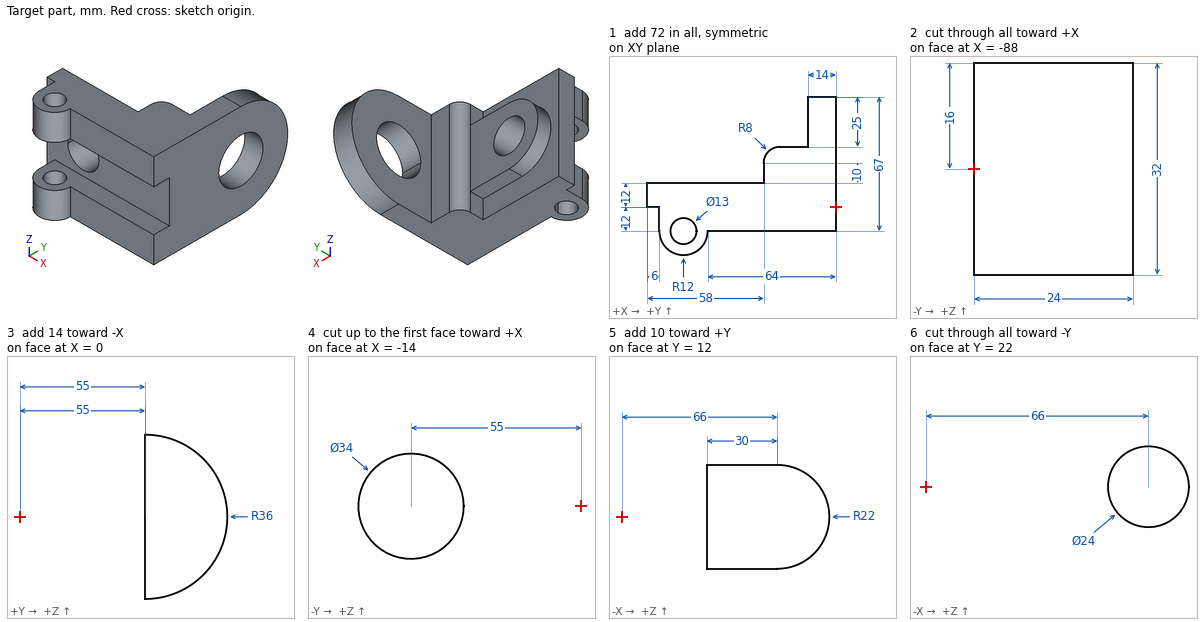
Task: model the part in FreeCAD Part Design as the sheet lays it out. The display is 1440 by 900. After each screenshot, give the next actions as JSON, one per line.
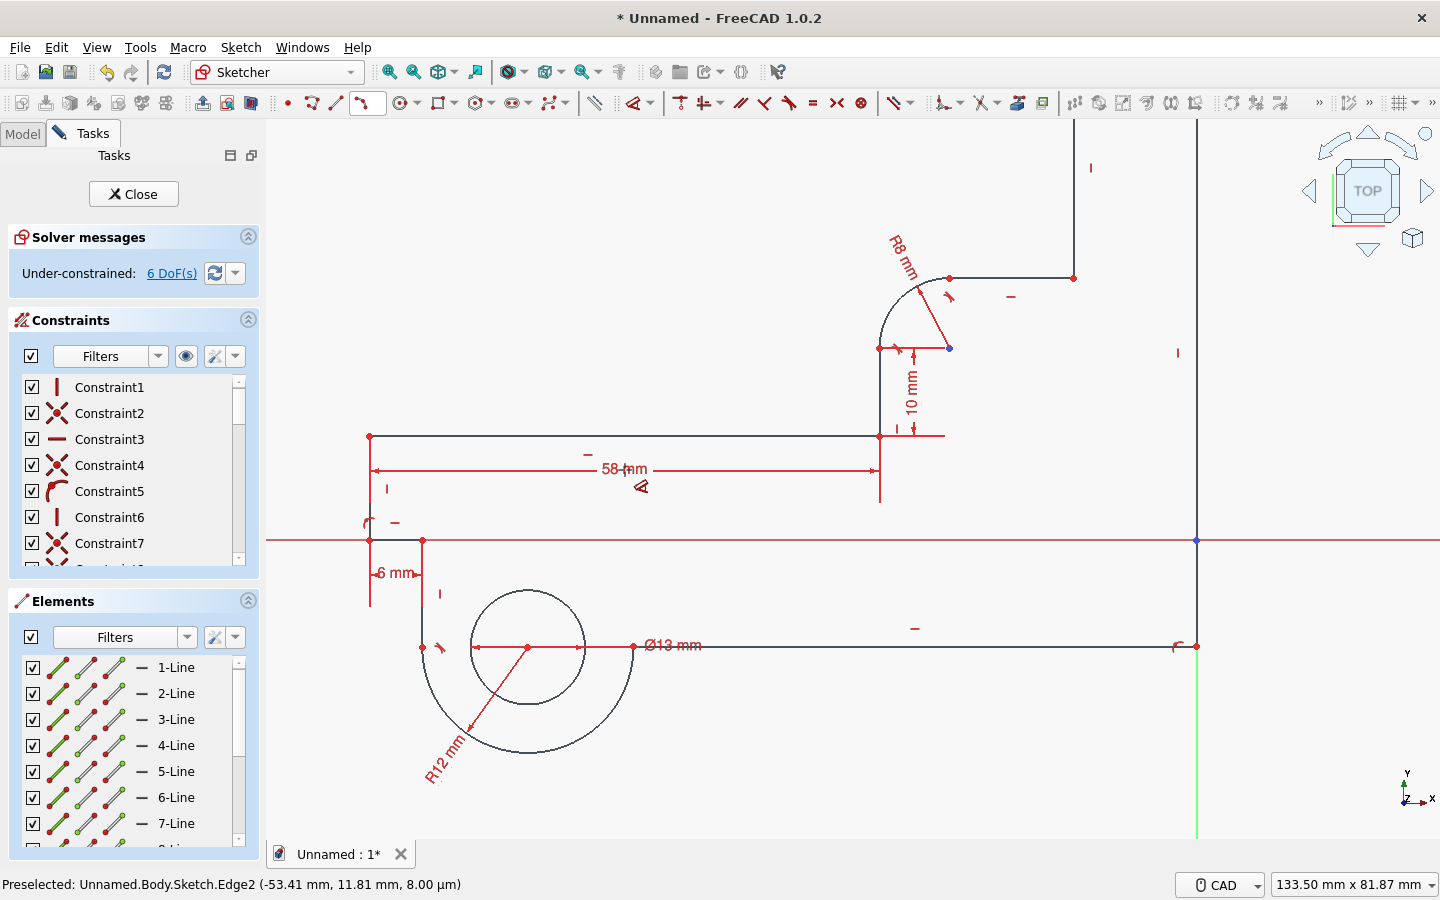
{"action": "left_click", "coordinate": [370, 468]}
{"action": "left_click", "coordinate": [336, 488]}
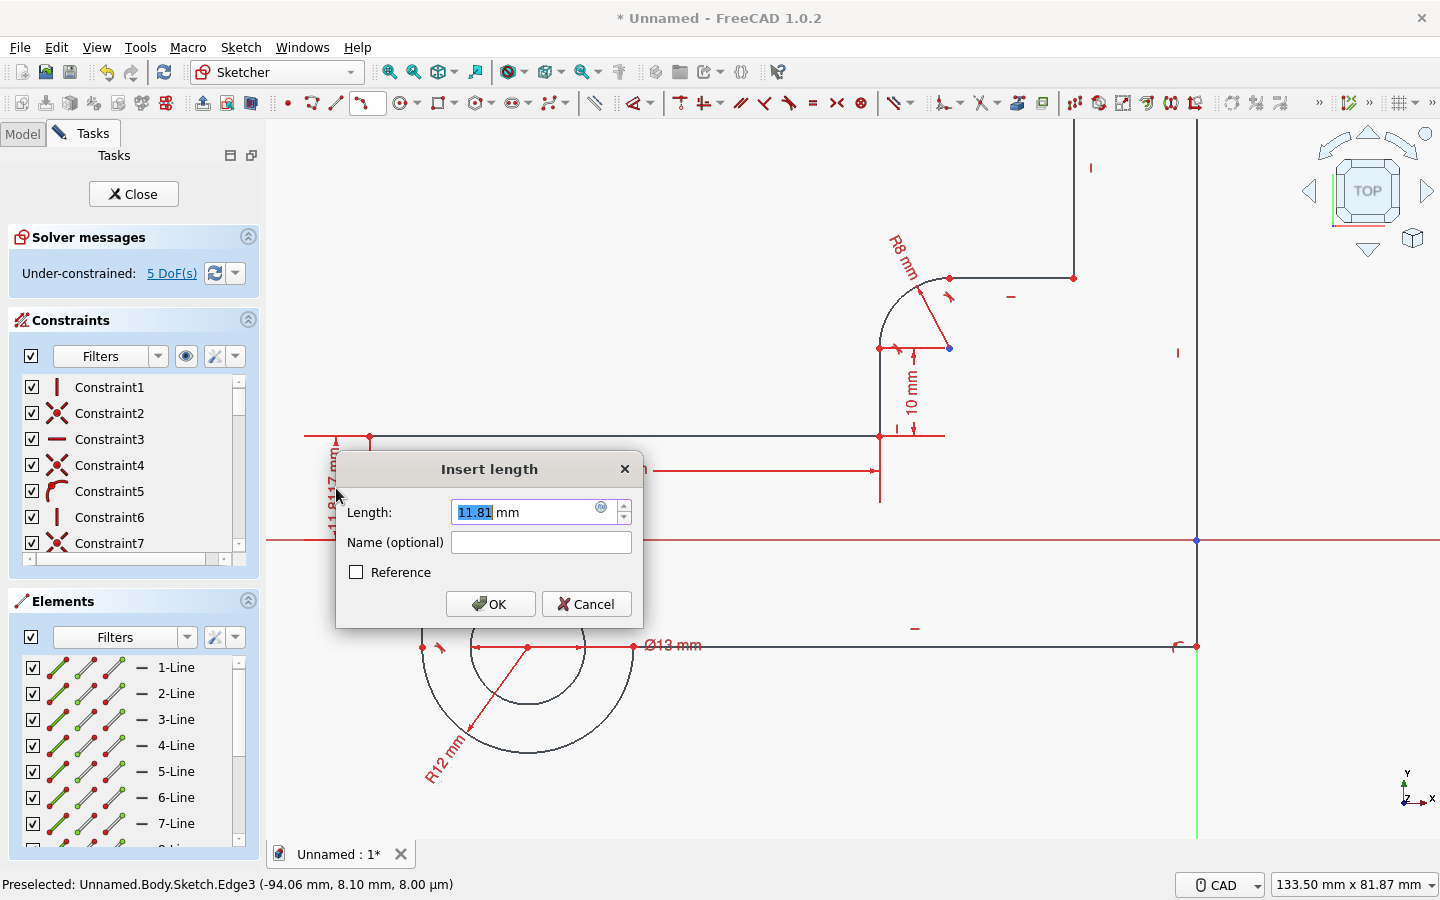
{"action": "type", "text": "12"}
{"action": "key", "text": "Return"}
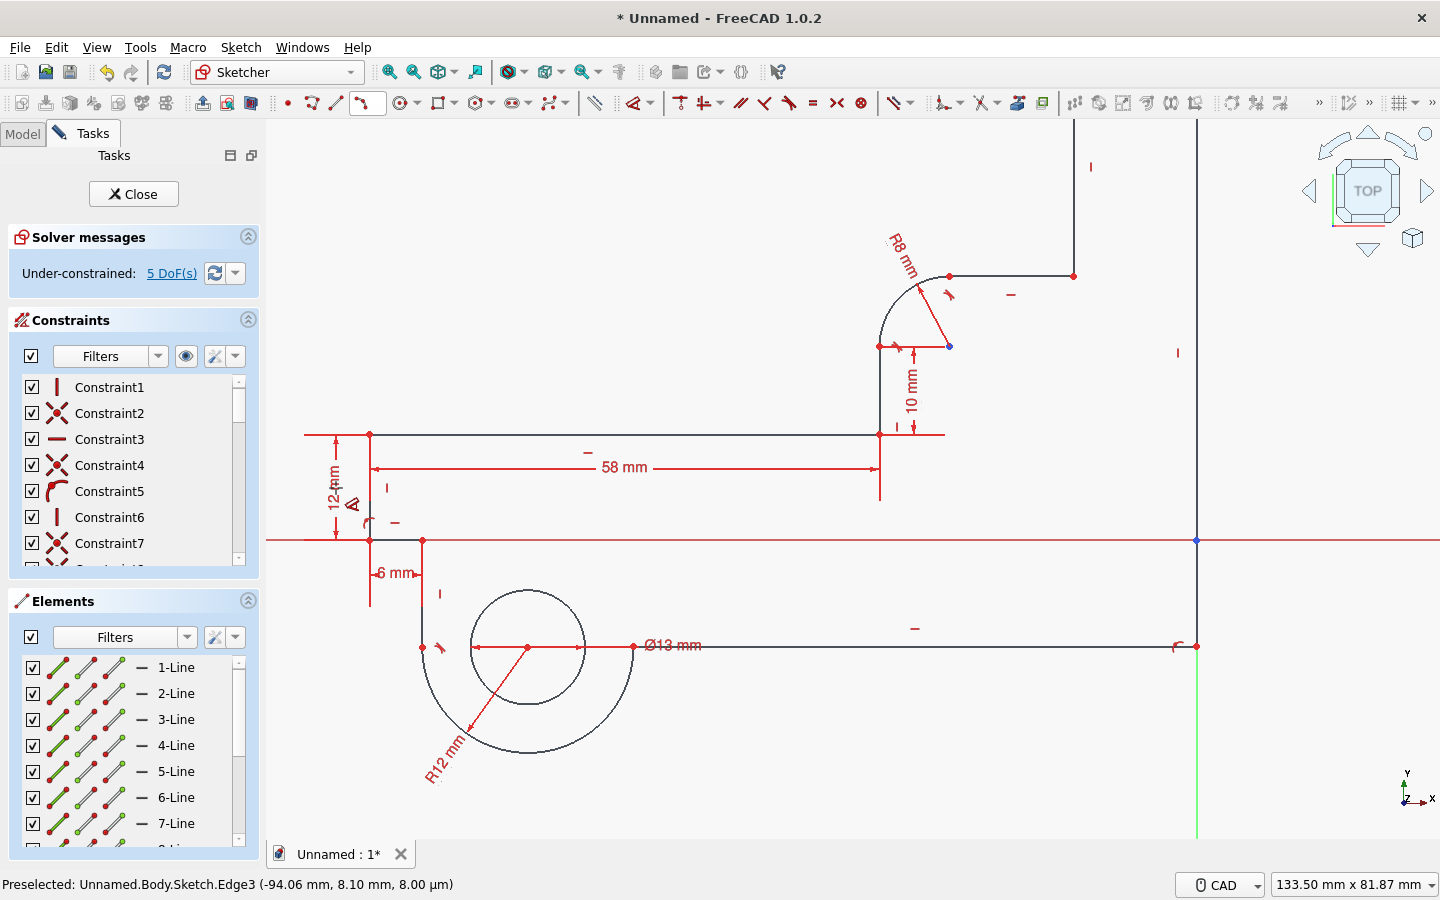
{"action": "left_click", "coordinate": [422, 572]}
{"action": "left_click", "coordinate": [388, 618]}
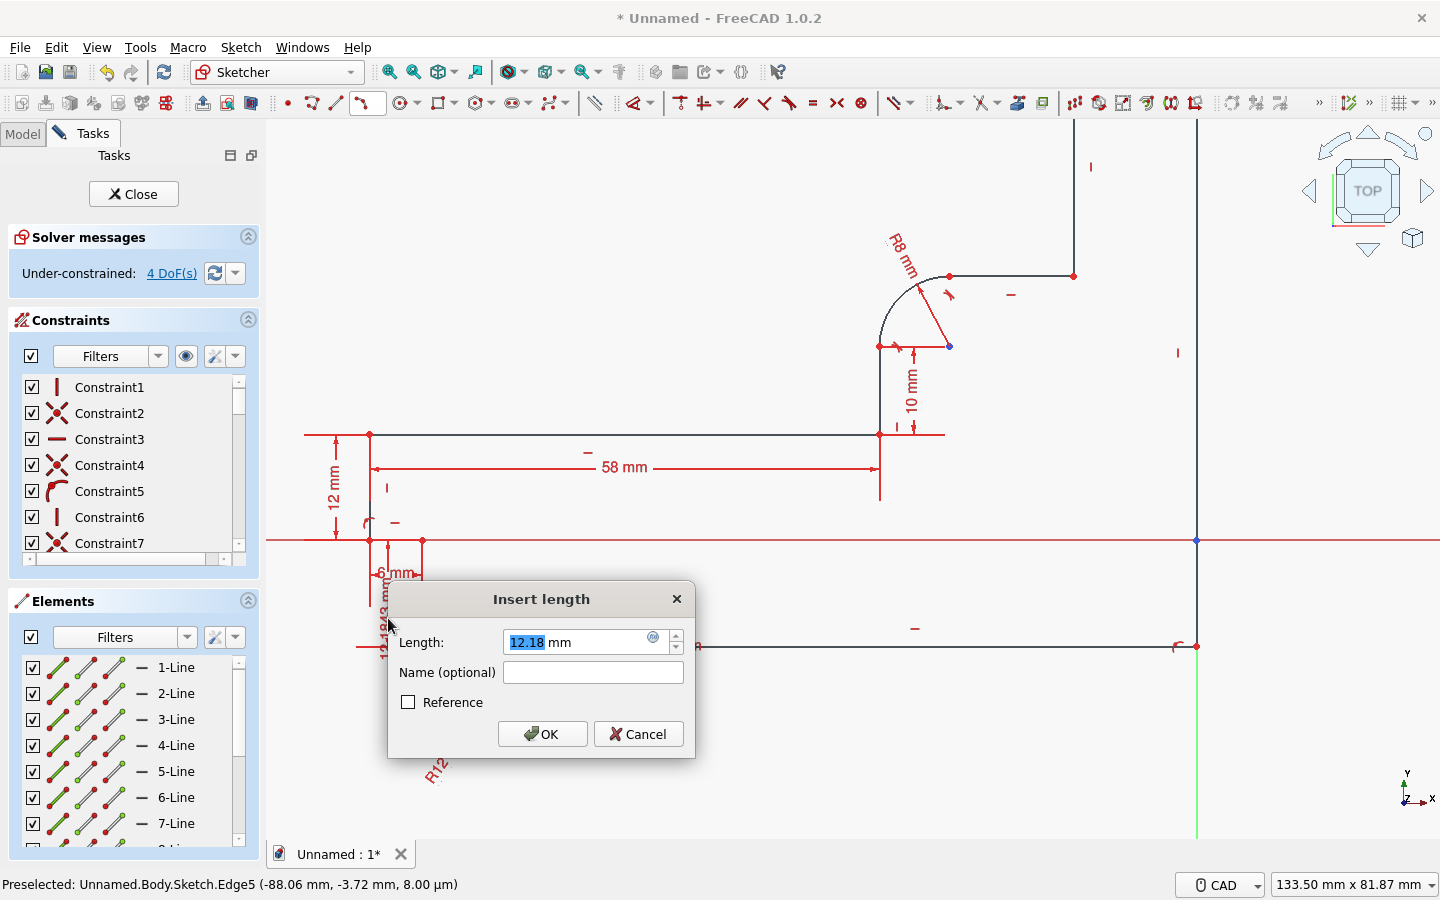
{"action": "type", "text": "12"}
{"action": "key", "text": "Return"}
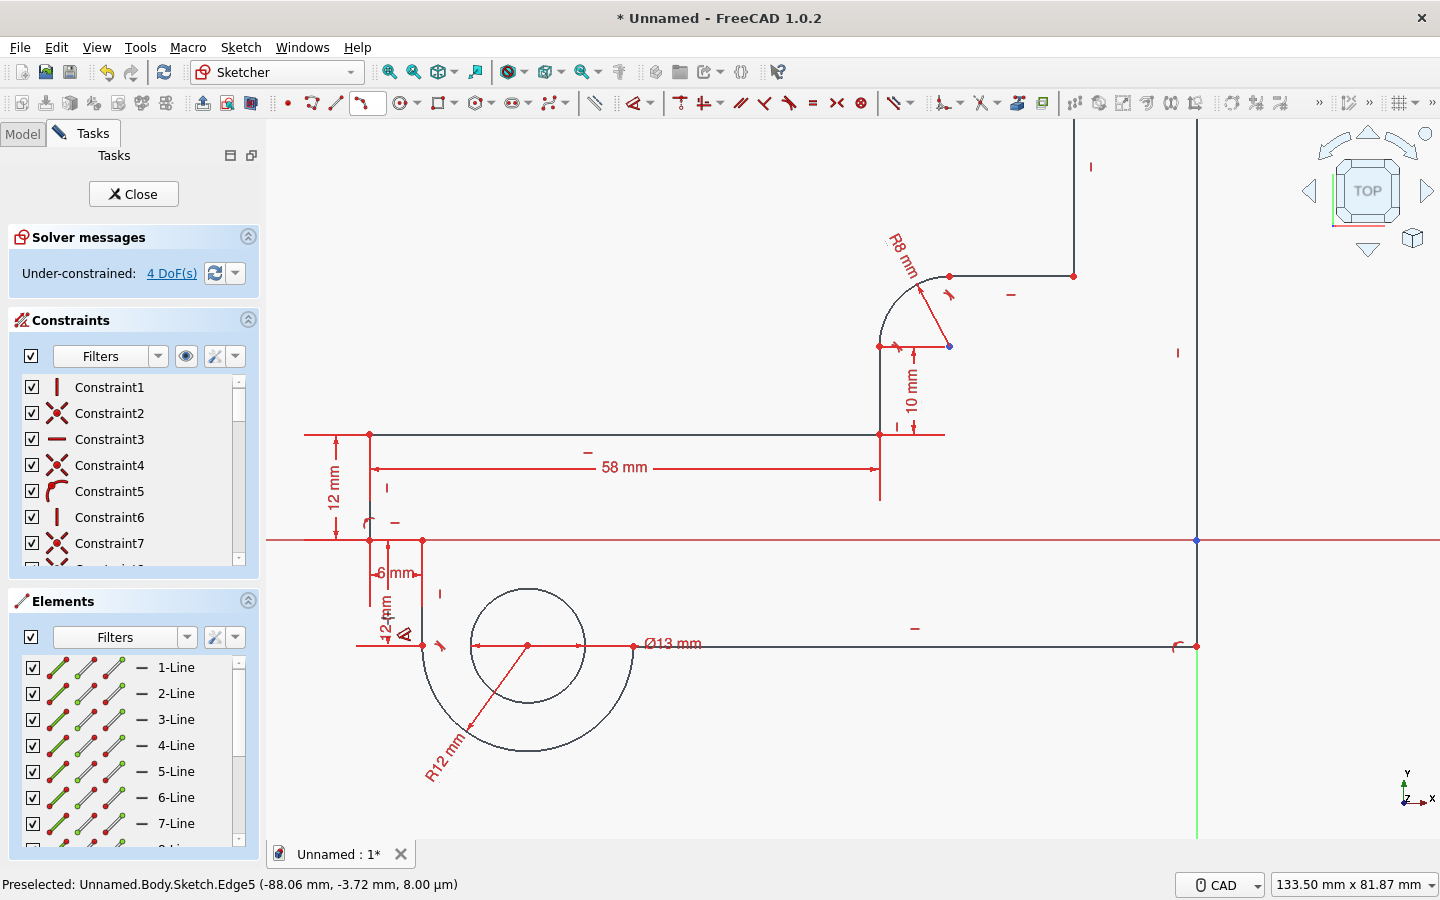
{"action": "left_click", "coordinate": [802, 647]}
{"action": "left_click", "coordinate": [915, 681]}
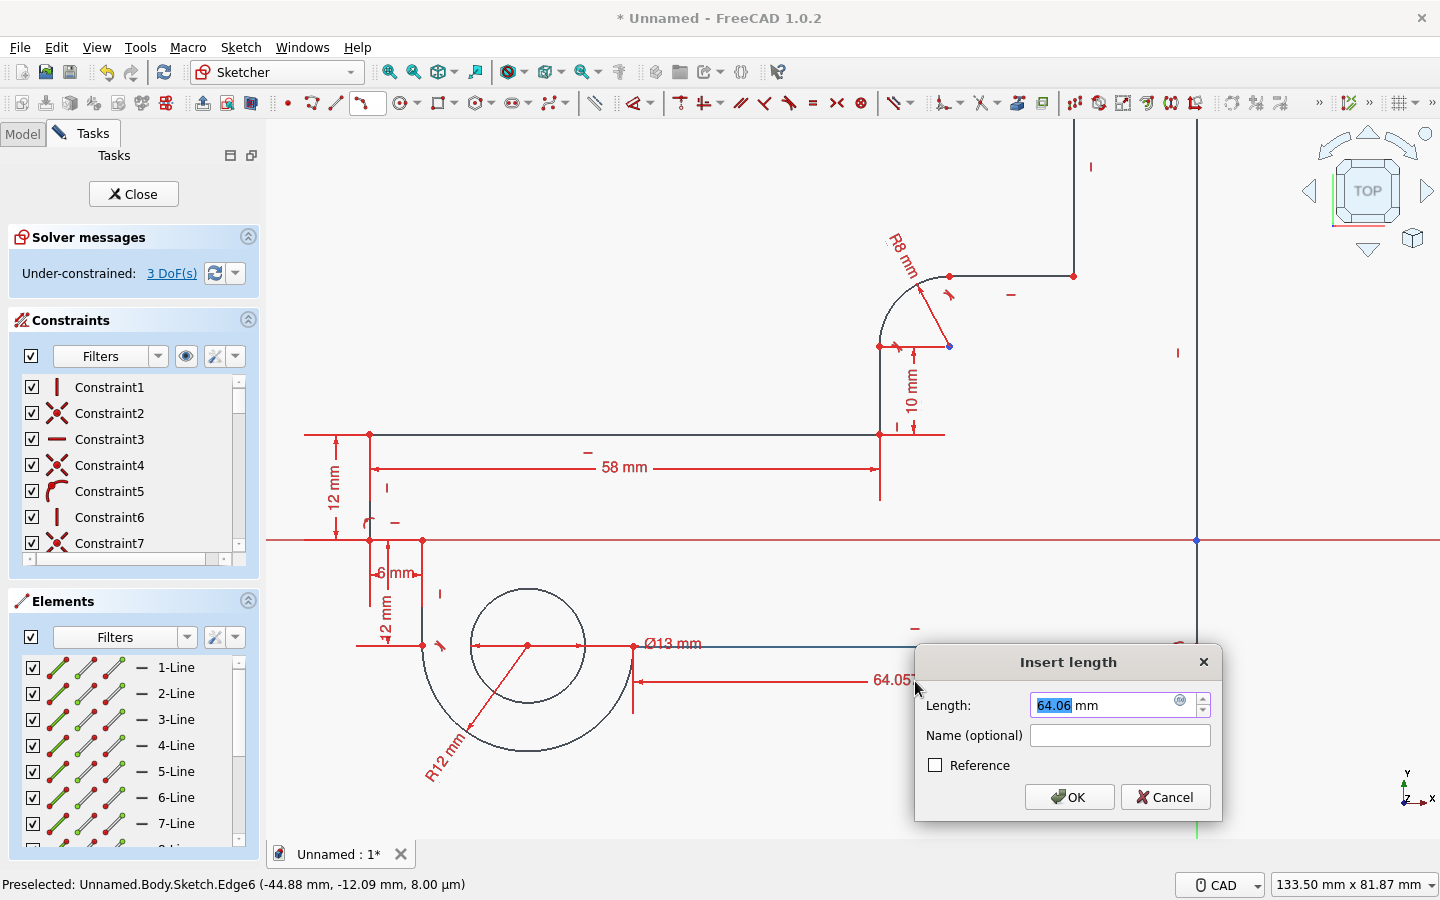
{"action": "type", "text": "64"}
{"action": "key", "text": "Return"}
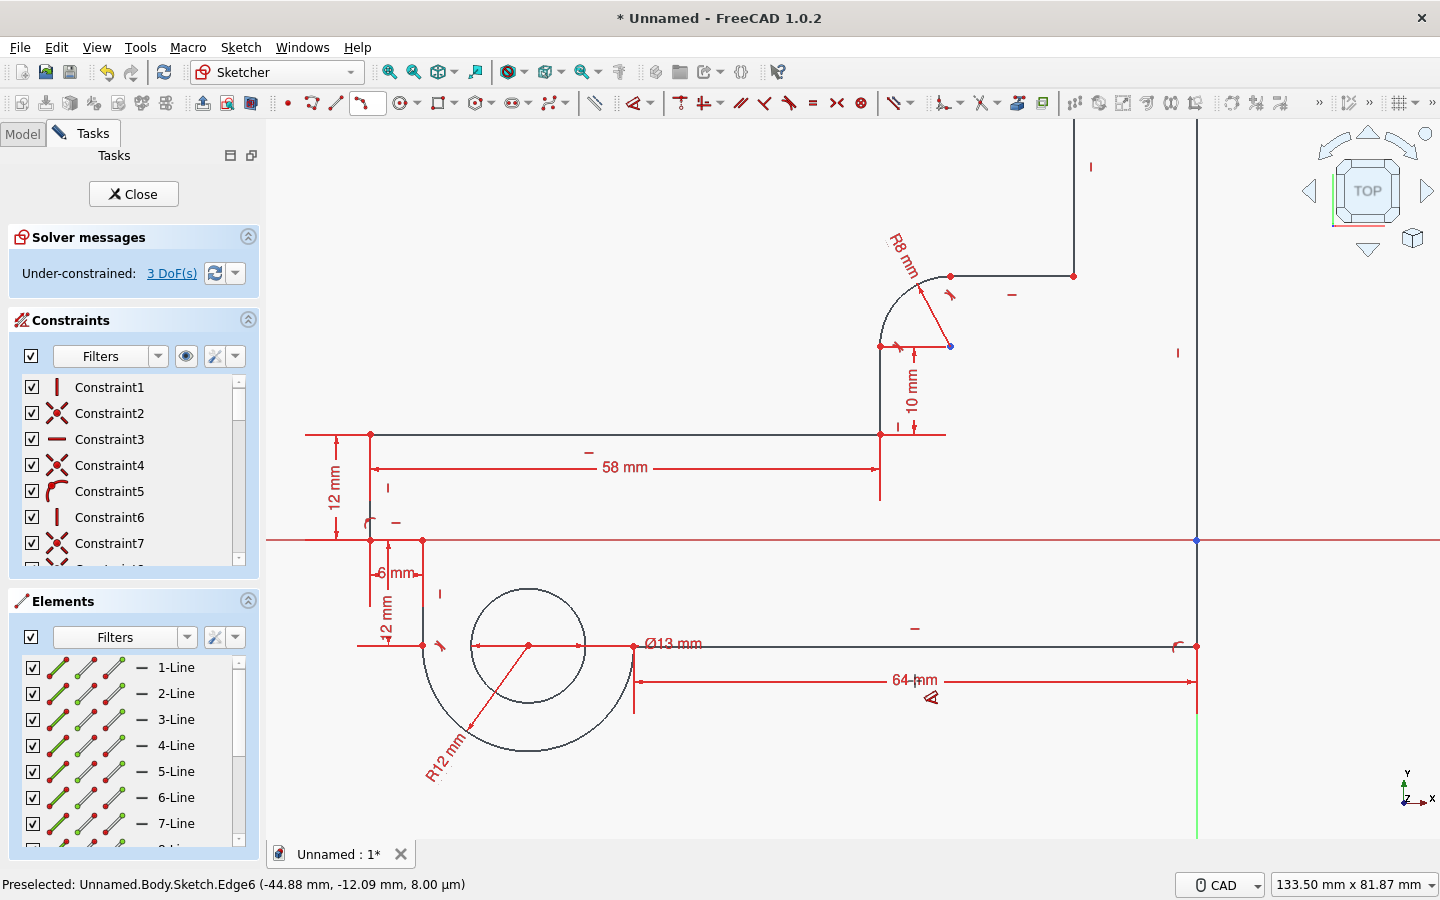
{"action": "left_click", "coordinate": [1197, 470]}
{"action": "left_click", "coordinate": [1231, 397]}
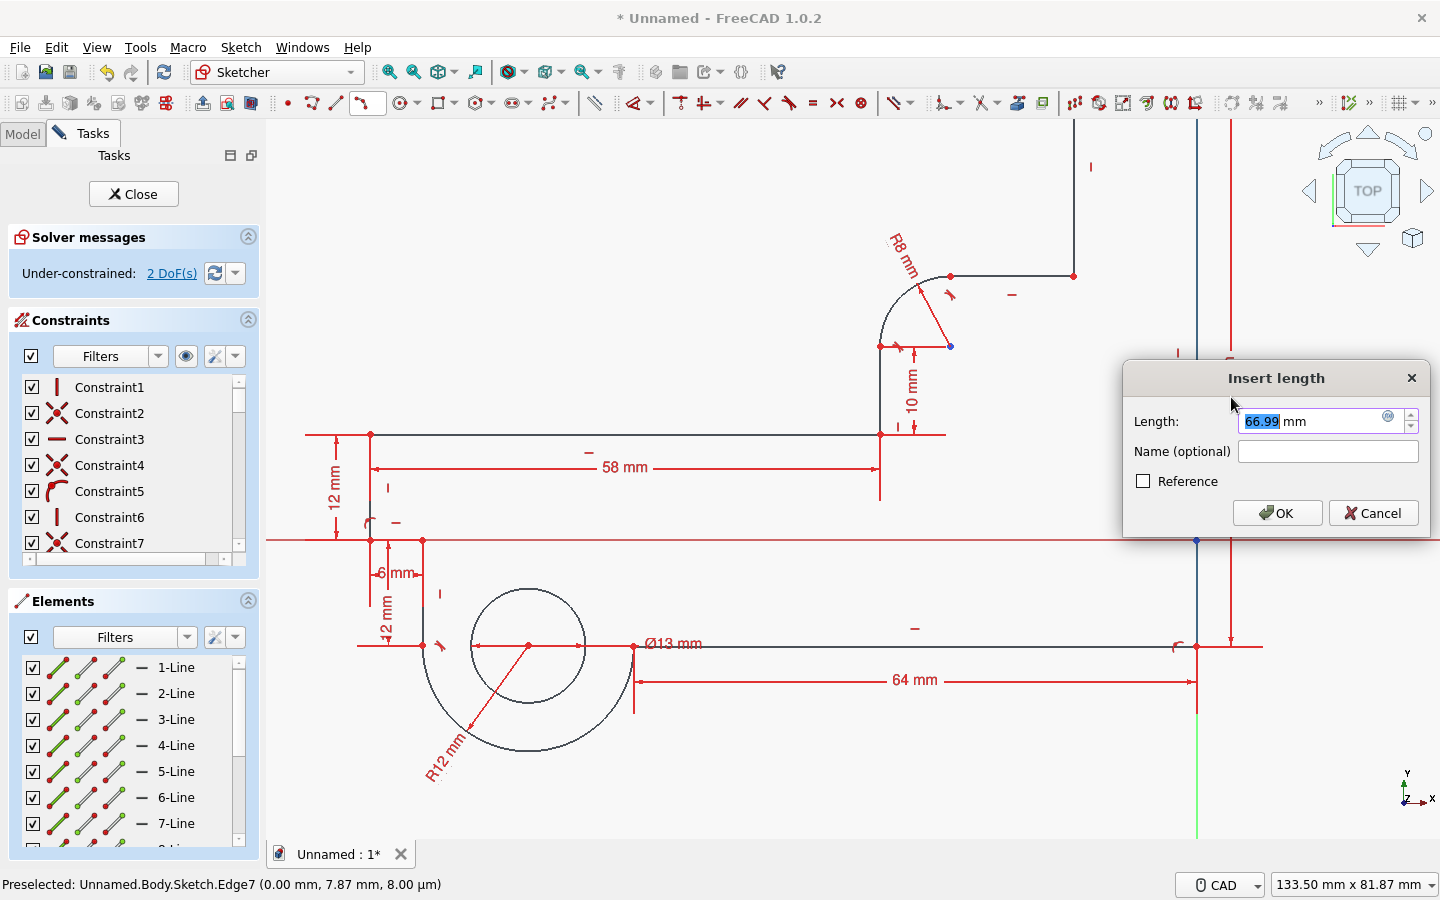
{"action": "type", "text": "67"}
{"action": "key", "text": "Return"}